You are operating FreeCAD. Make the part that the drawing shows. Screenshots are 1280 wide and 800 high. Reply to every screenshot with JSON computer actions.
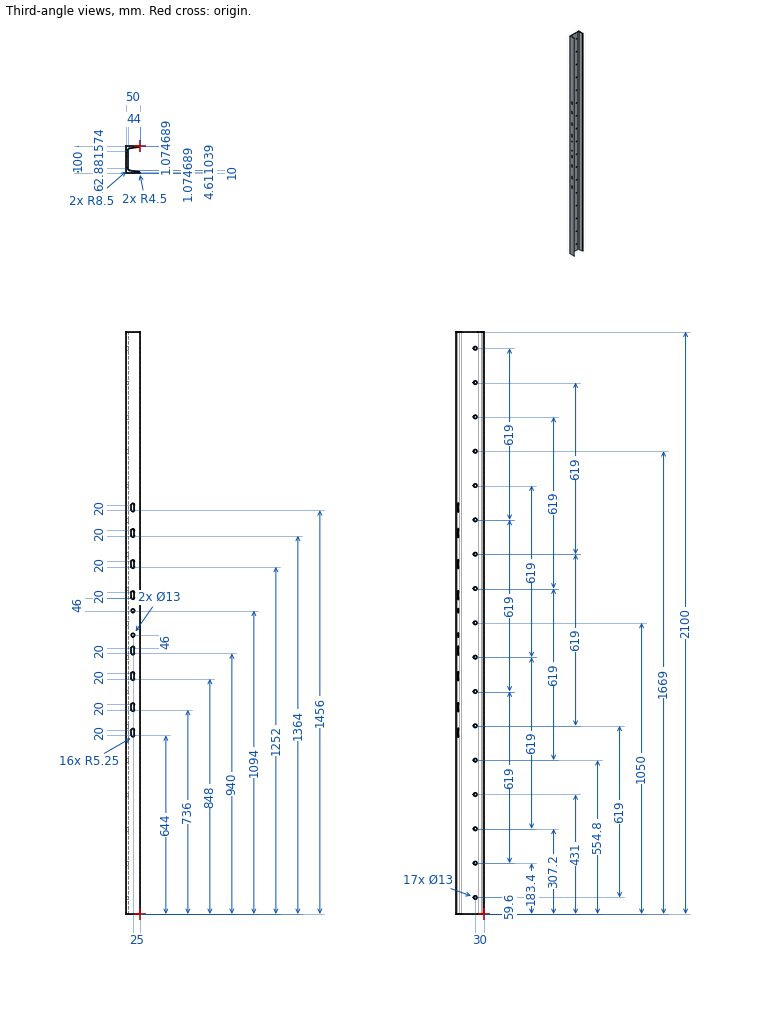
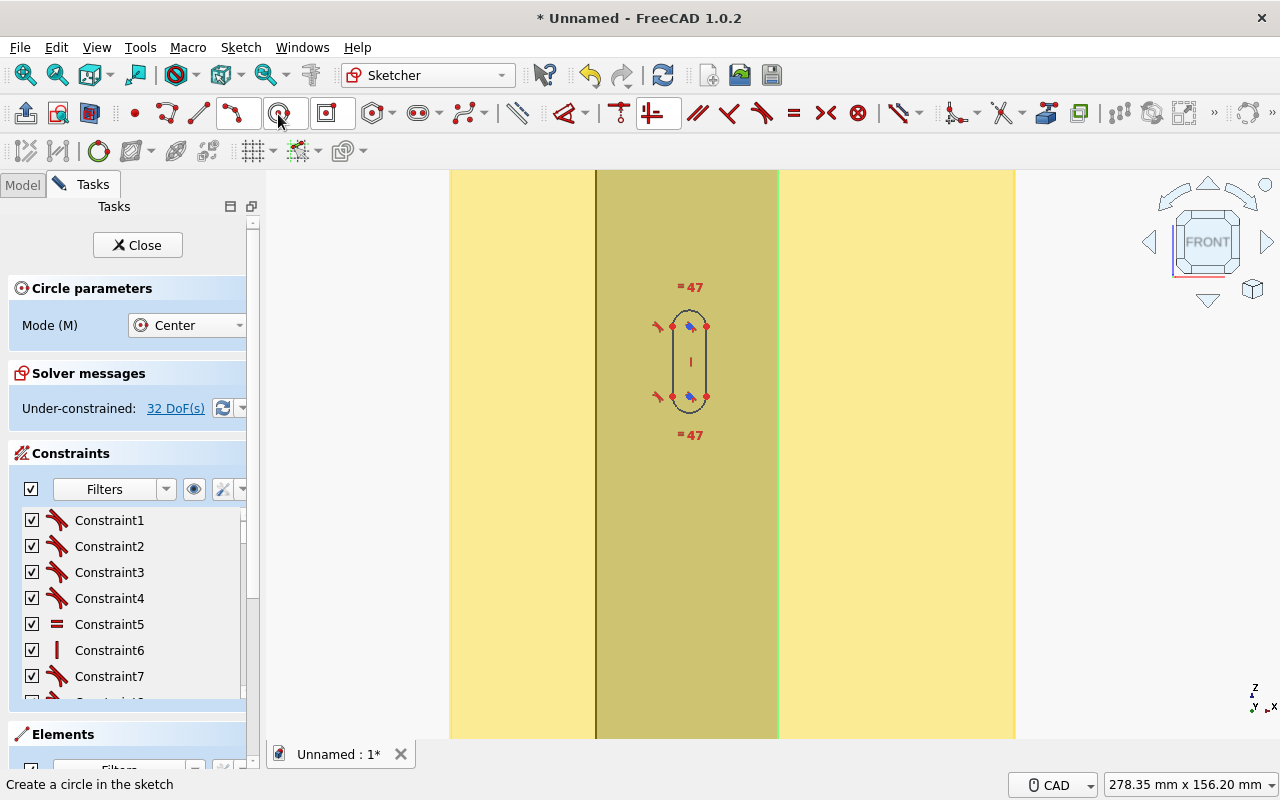
{"action": "scroll", "coordinate": [703, 364], "scroll_direction": "down", "scroll_amount": 14}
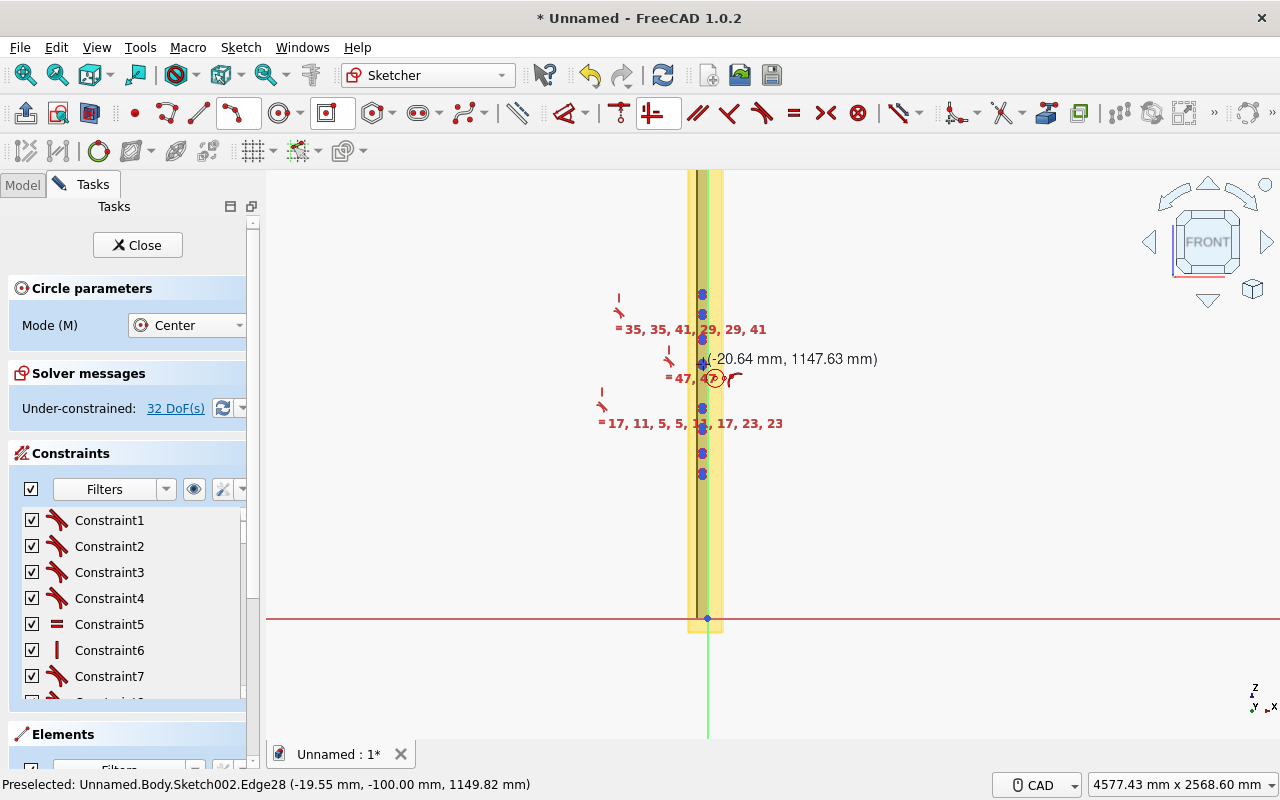
{"action": "scroll", "coordinate": [702, 396], "scroll_direction": "up", "scroll_amount": 14}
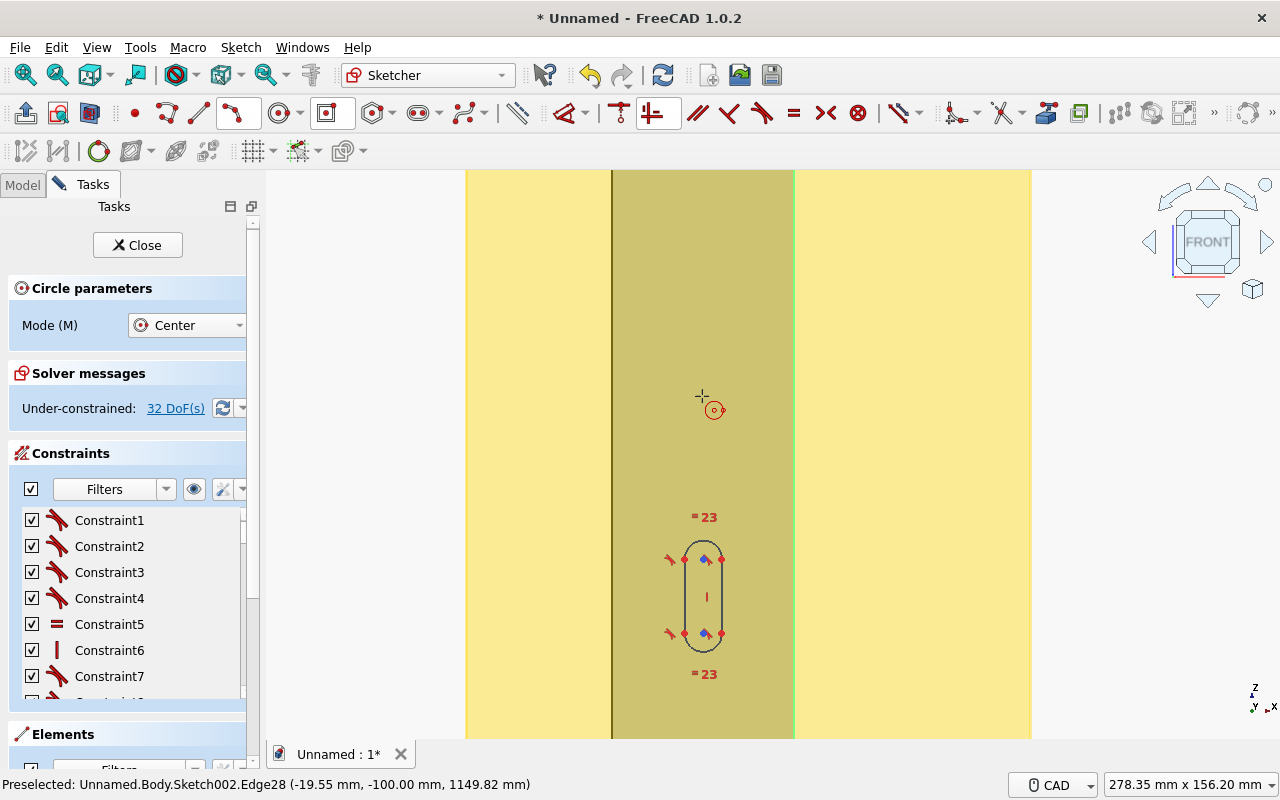
{"action": "scroll", "coordinate": [702, 396], "scroll_direction": "down", "scroll_amount": 14}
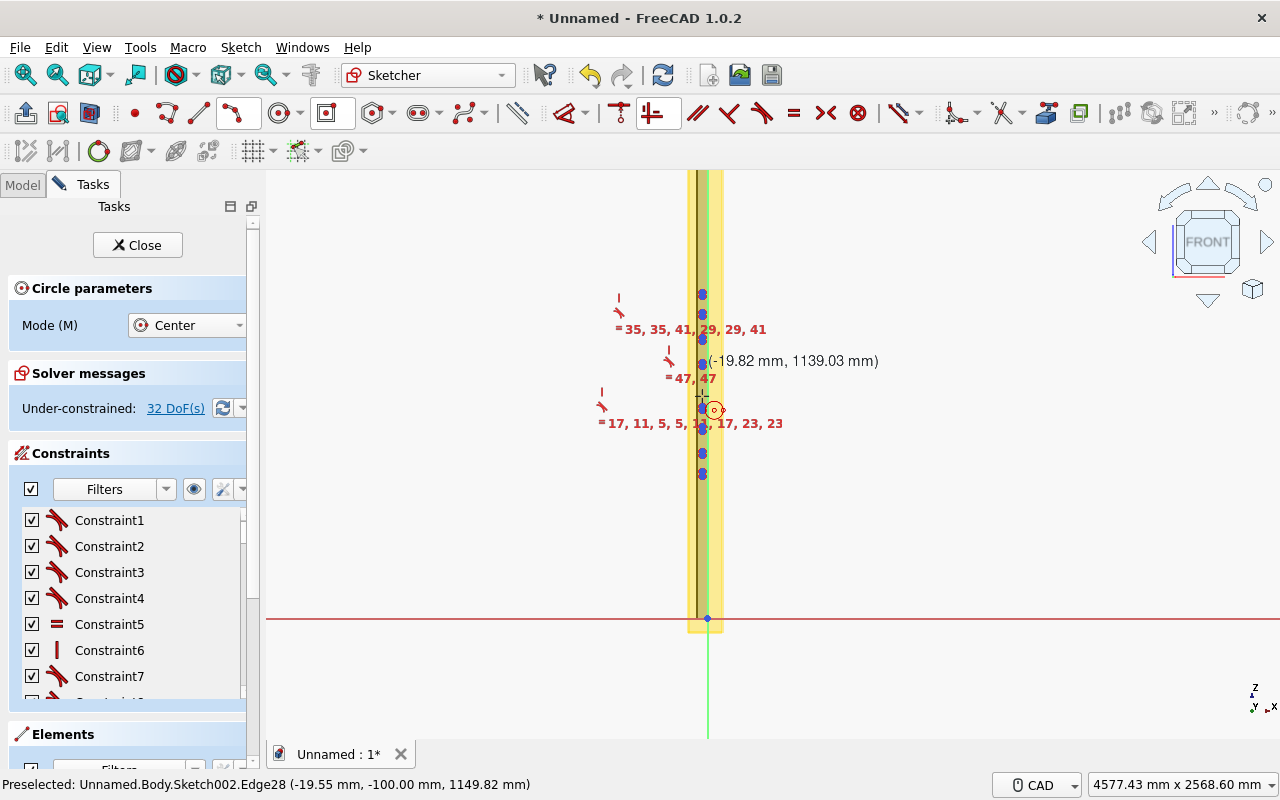
{"action": "scroll", "coordinate": [702, 396], "scroll_direction": "up", "scroll_amount": 6}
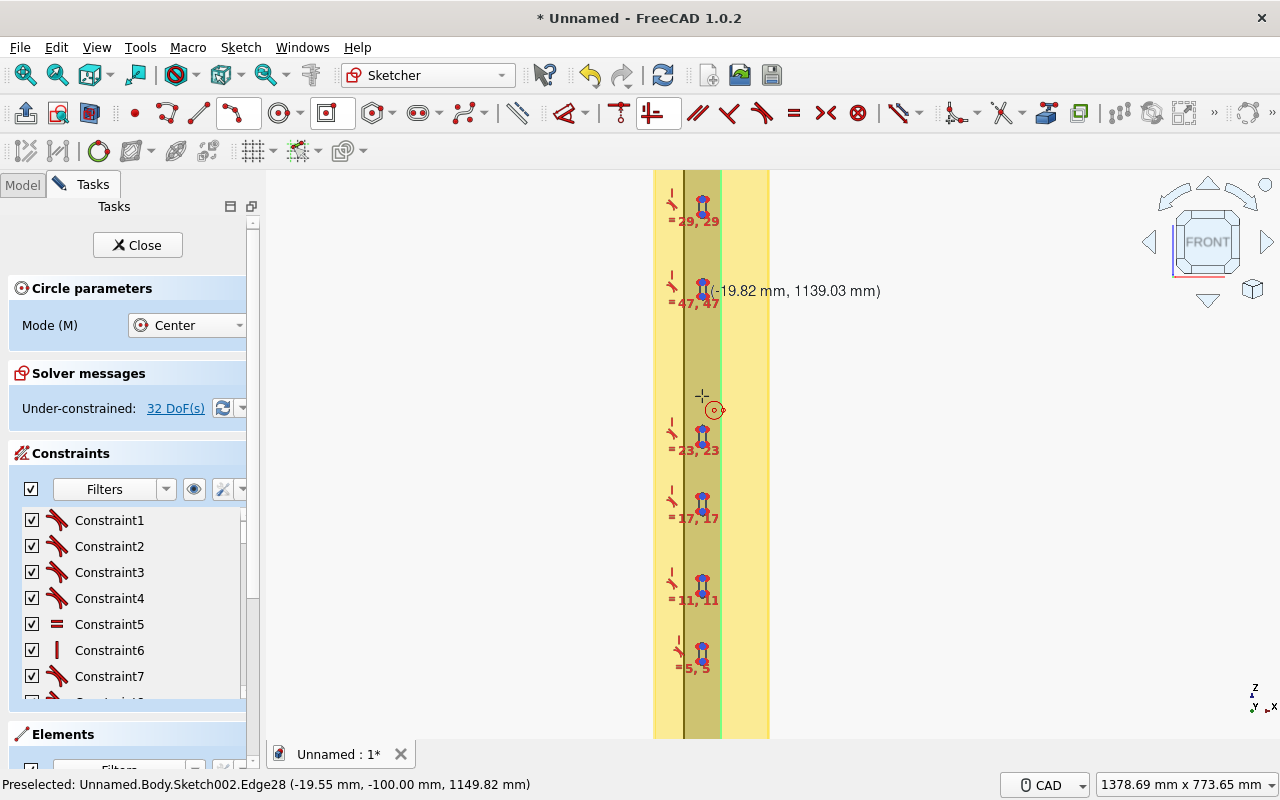
{"action": "left_click", "coordinate": [702, 394]}
{"action": "mouse_move", "coordinate": [706, 391]}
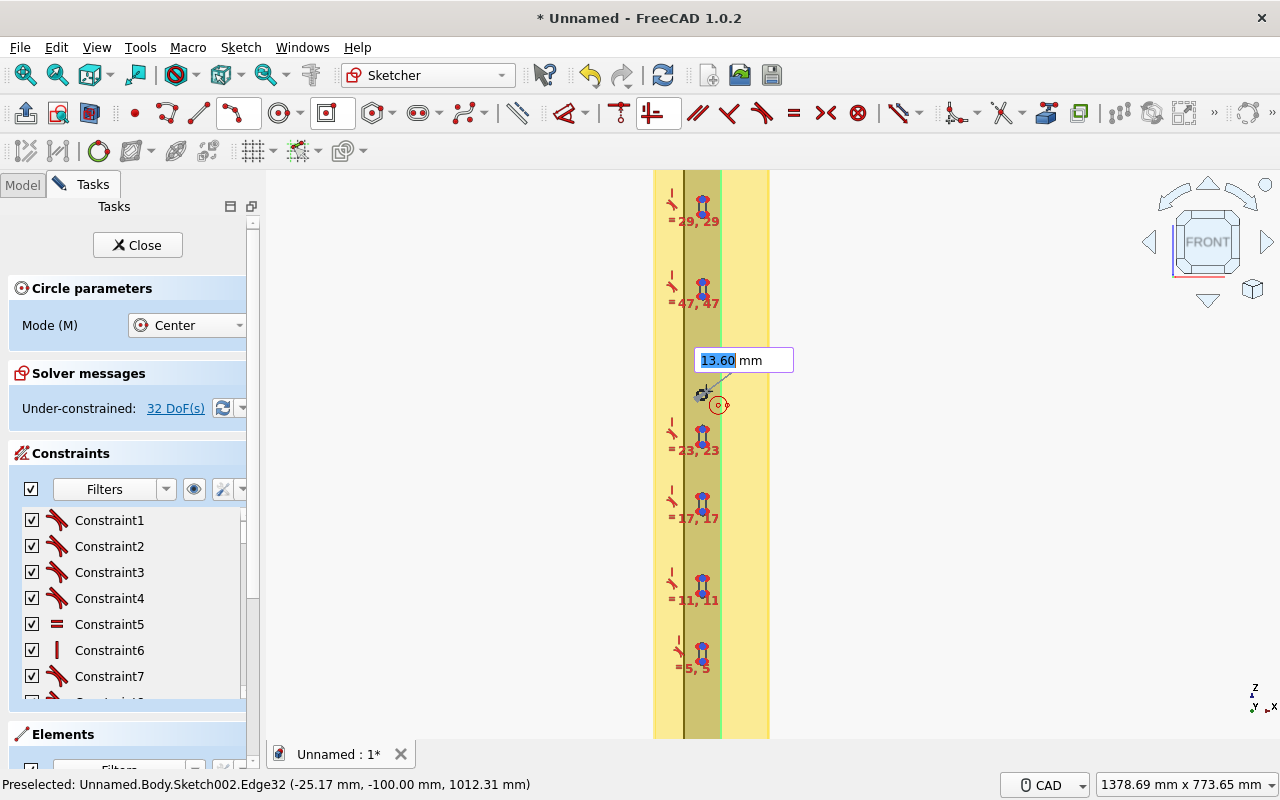
{"action": "type", "text": "13"}
{"action": "key", "text": "Return"}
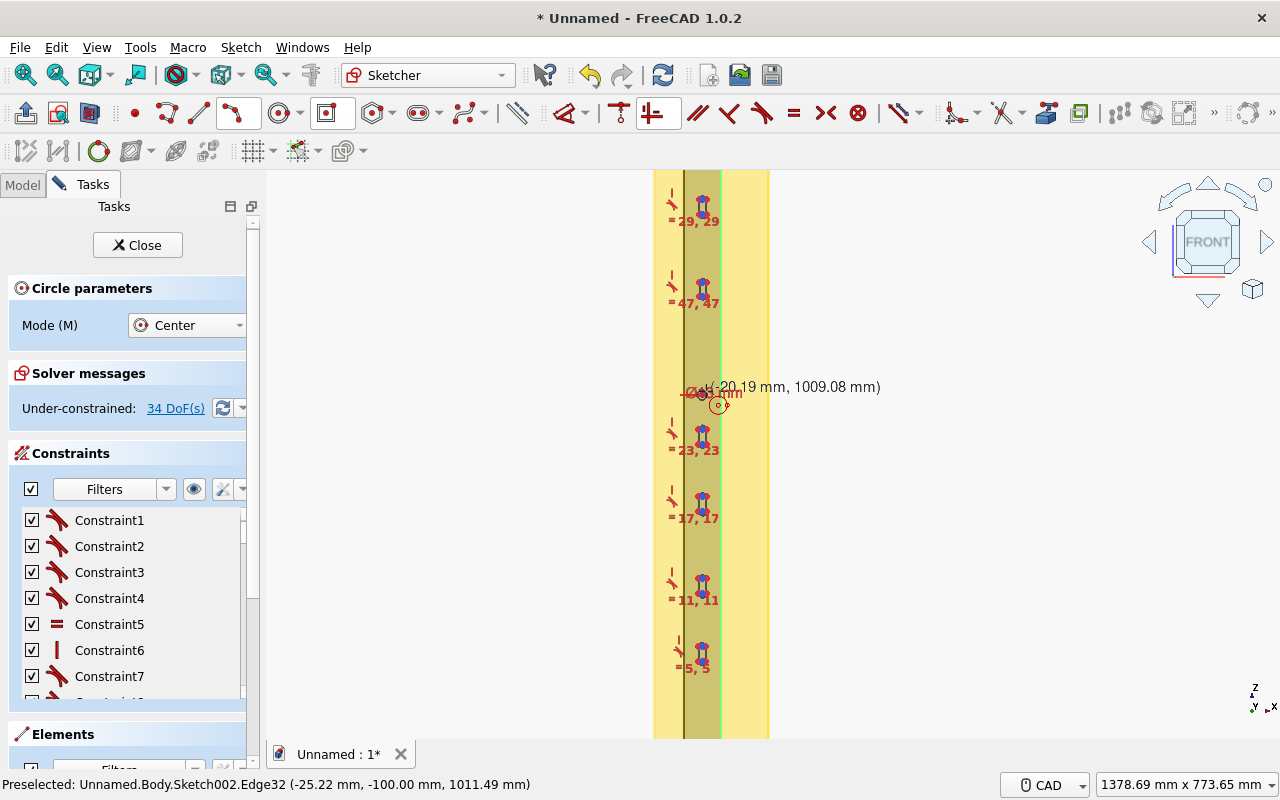
{"action": "scroll", "coordinate": [702, 330], "scroll_direction": "up", "scroll_amount": 8}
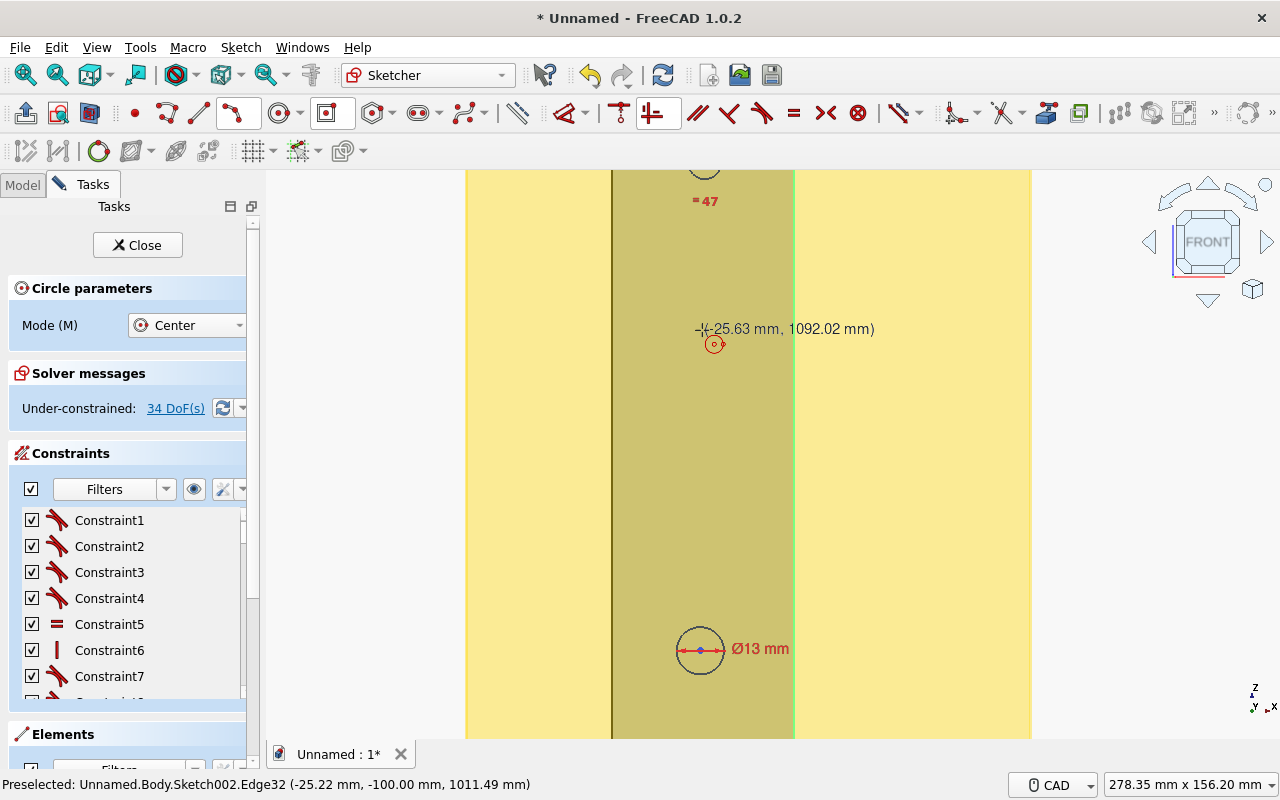
{"action": "scroll", "coordinate": [702, 379], "scroll_direction": "down", "scroll_amount": 14}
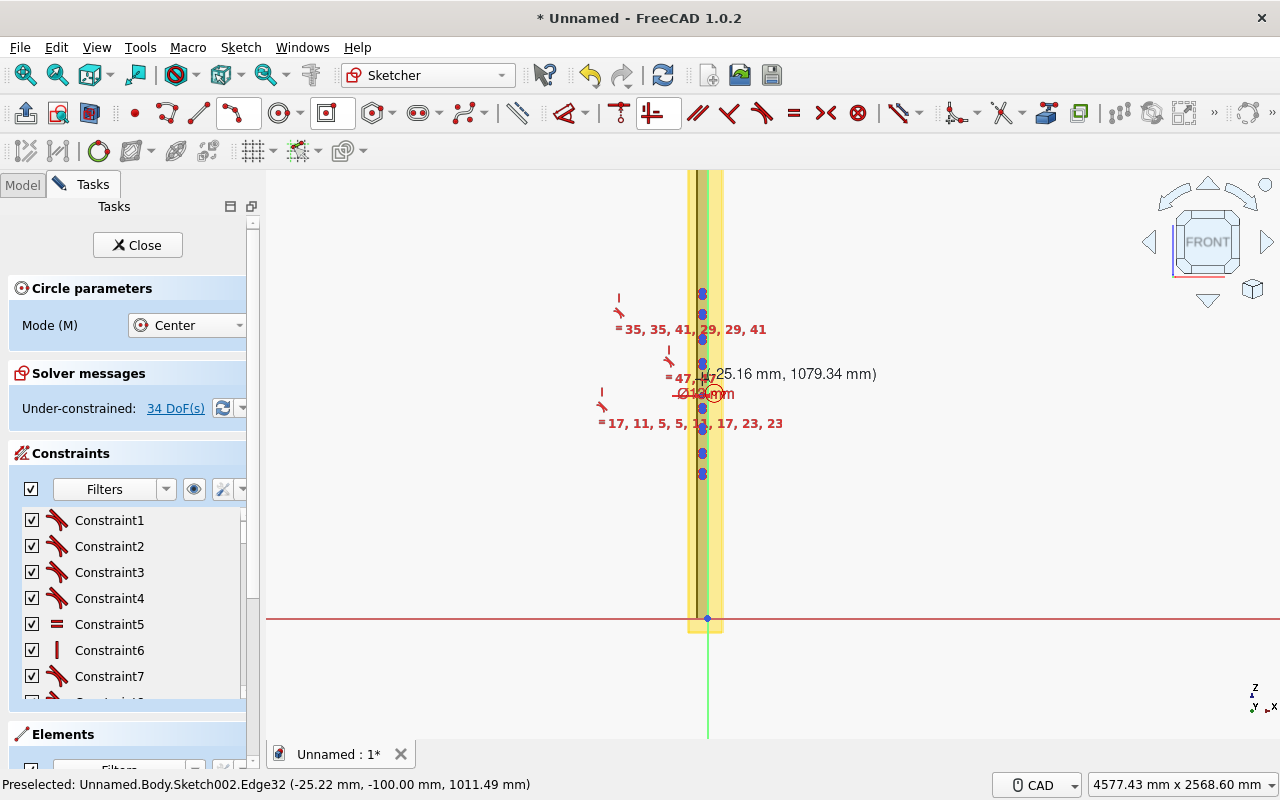
{"action": "scroll", "coordinate": [702, 376], "scroll_direction": "up", "scroll_amount": 6}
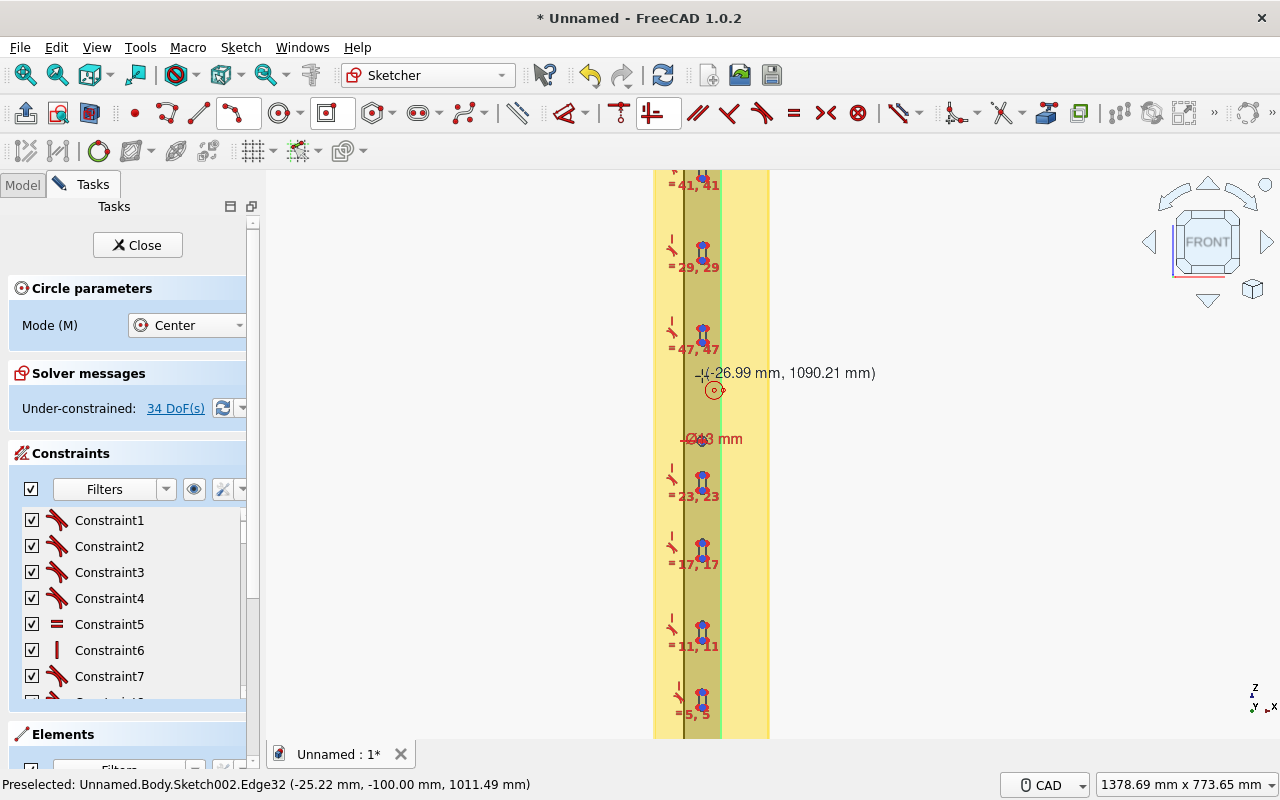
{"action": "left_click", "coordinate": [702, 376]}
{"action": "mouse_move", "coordinate": [706, 372]}